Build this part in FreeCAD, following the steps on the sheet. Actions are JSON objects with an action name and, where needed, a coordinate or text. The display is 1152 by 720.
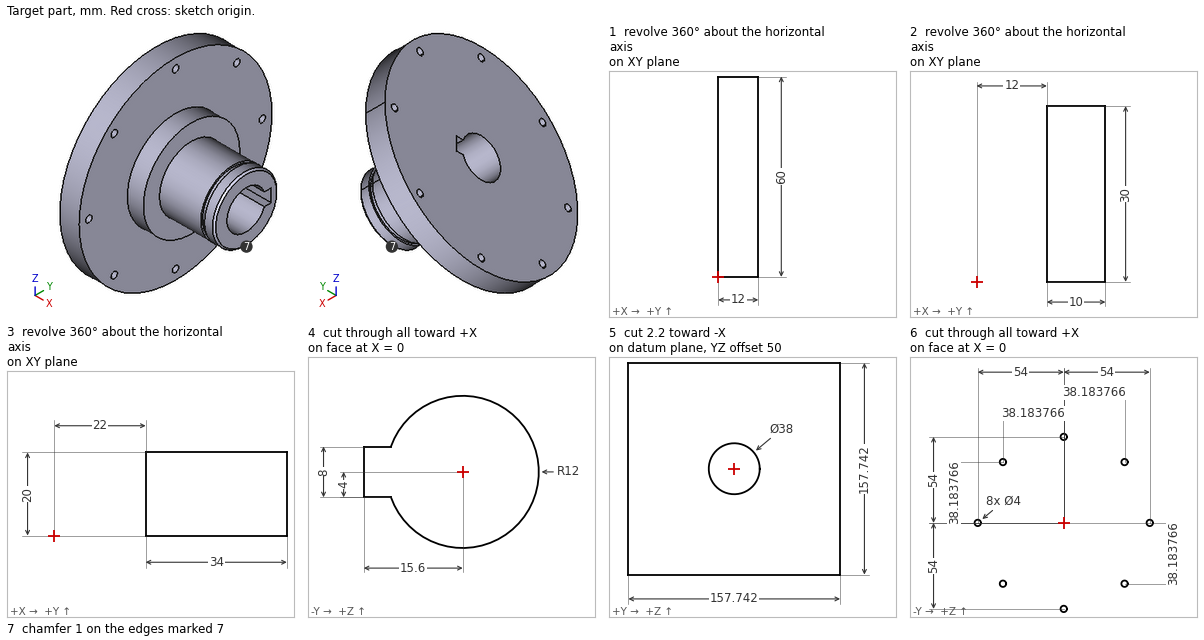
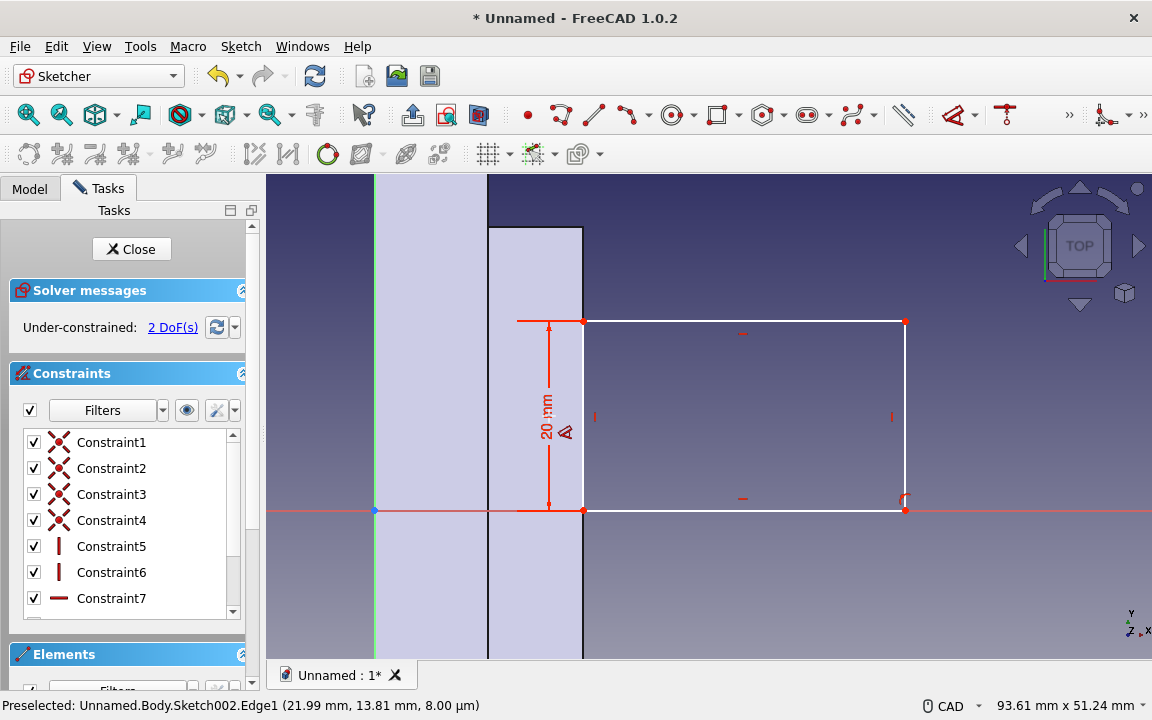
{"action": "left_click", "coordinate": [680, 511]}
{"action": "left_click", "coordinate": [744, 545]}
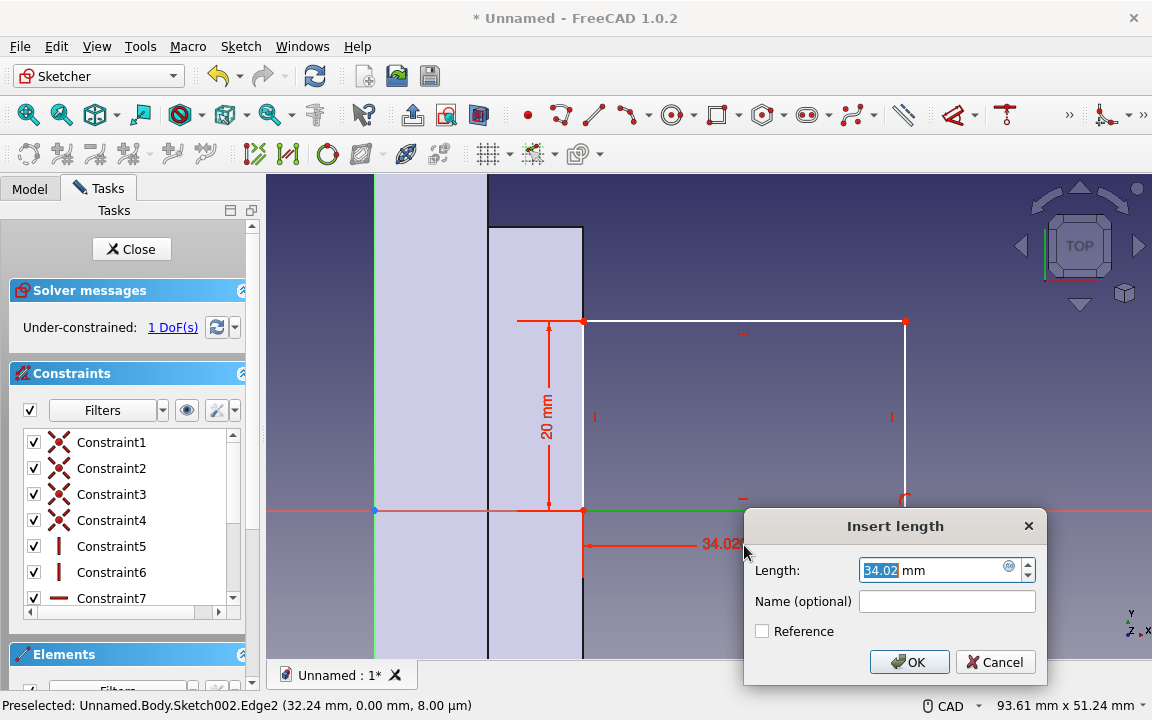
{"action": "type", "text": "34"}
{"action": "key", "text": "Return"}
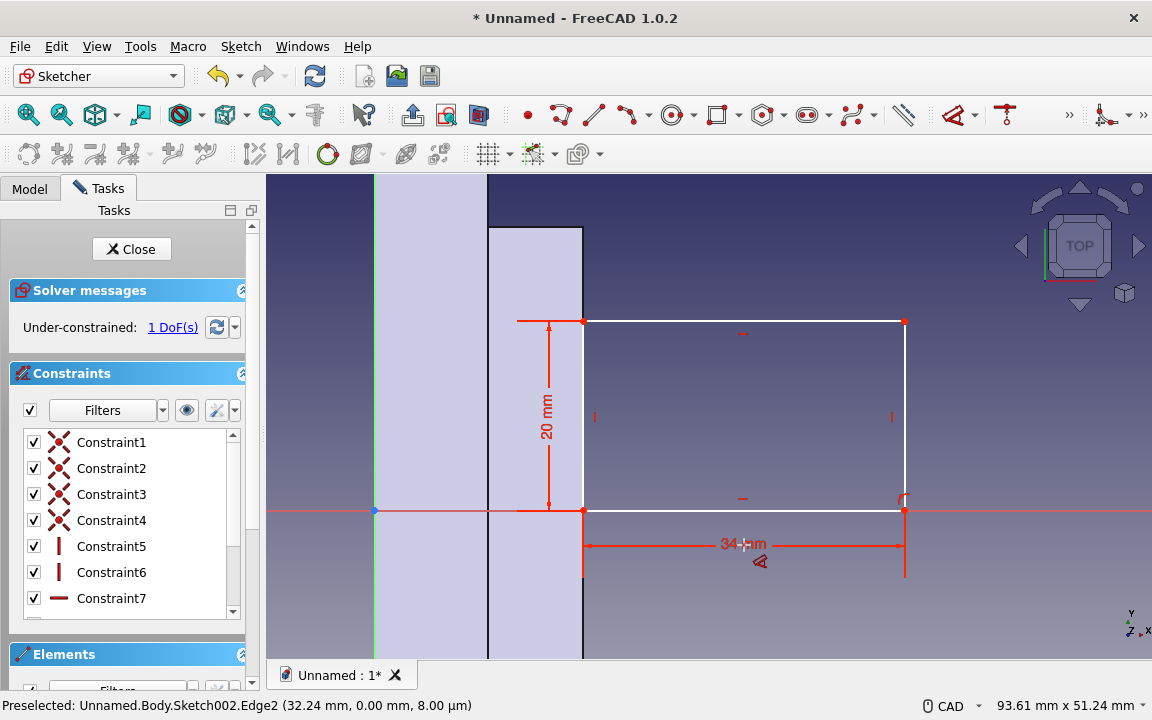
{"action": "left_click", "coordinate": [583, 321]}
{"action": "left_click", "coordinate": [479, 545]}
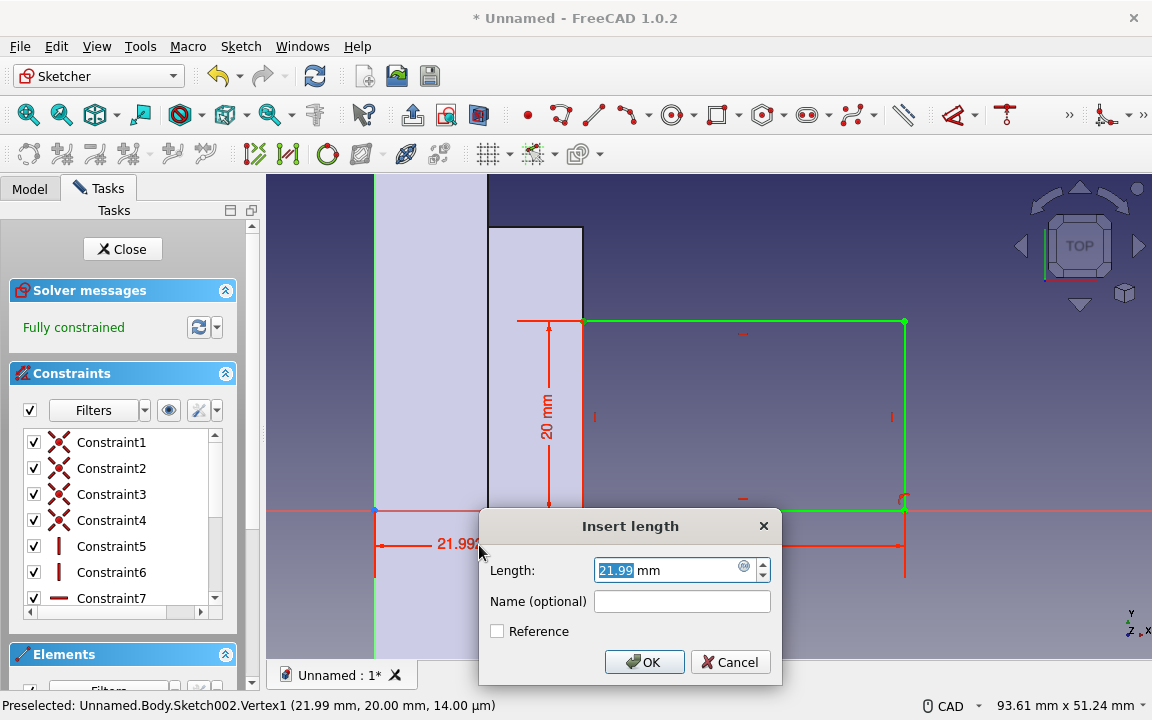
{"action": "type", "text": "22"}
{"action": "key", "text": "Return"}
{"action": "key", "text": "Escape"}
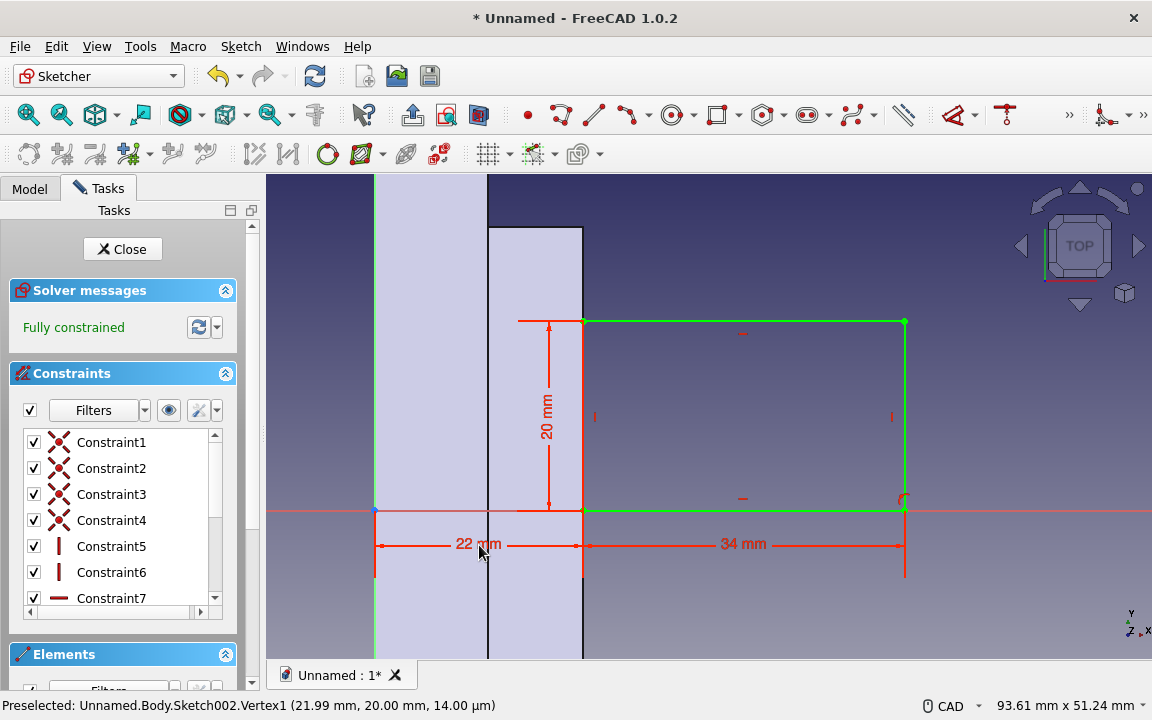
{"action": "left_click", "coordinate": [123, 249]}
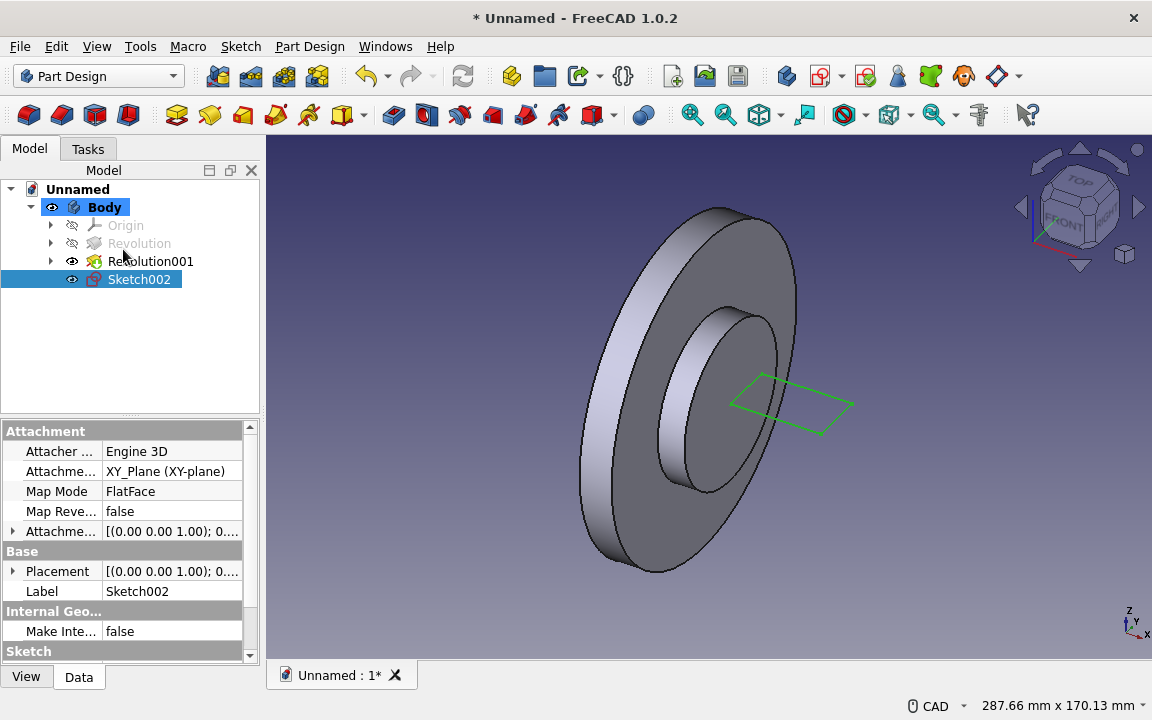
{"action": "left_click", "coordinate": [210, 116]}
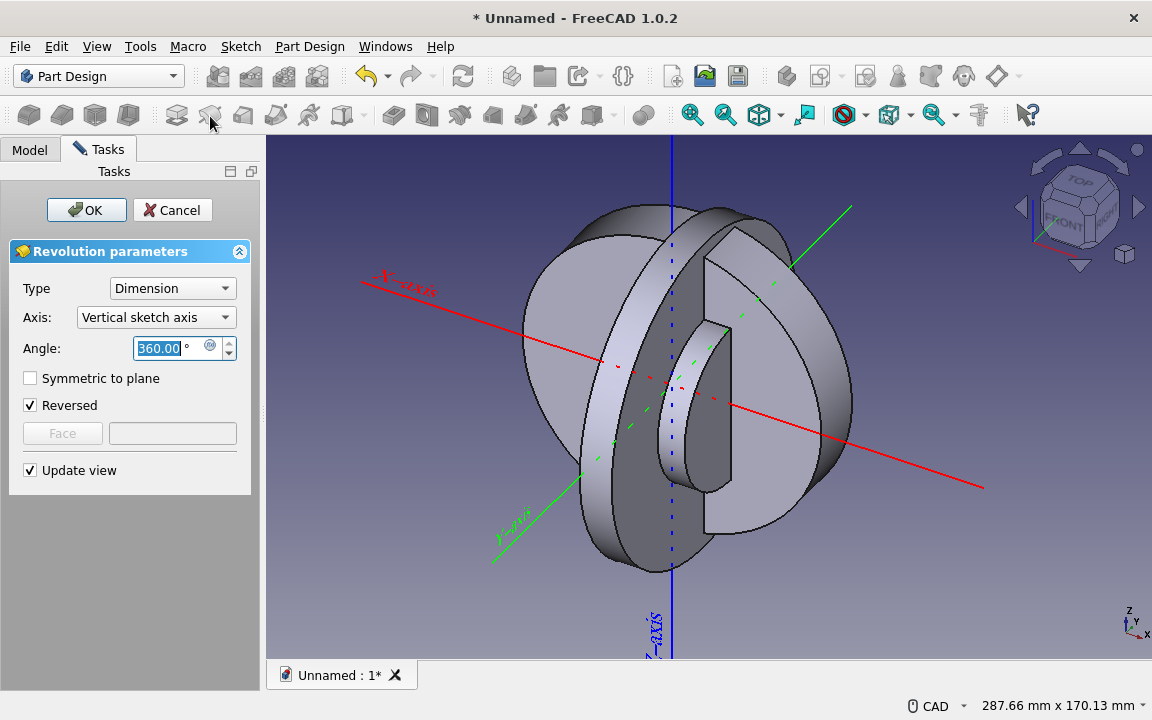
{"action": "left_click", "coordinate": [157, 318]}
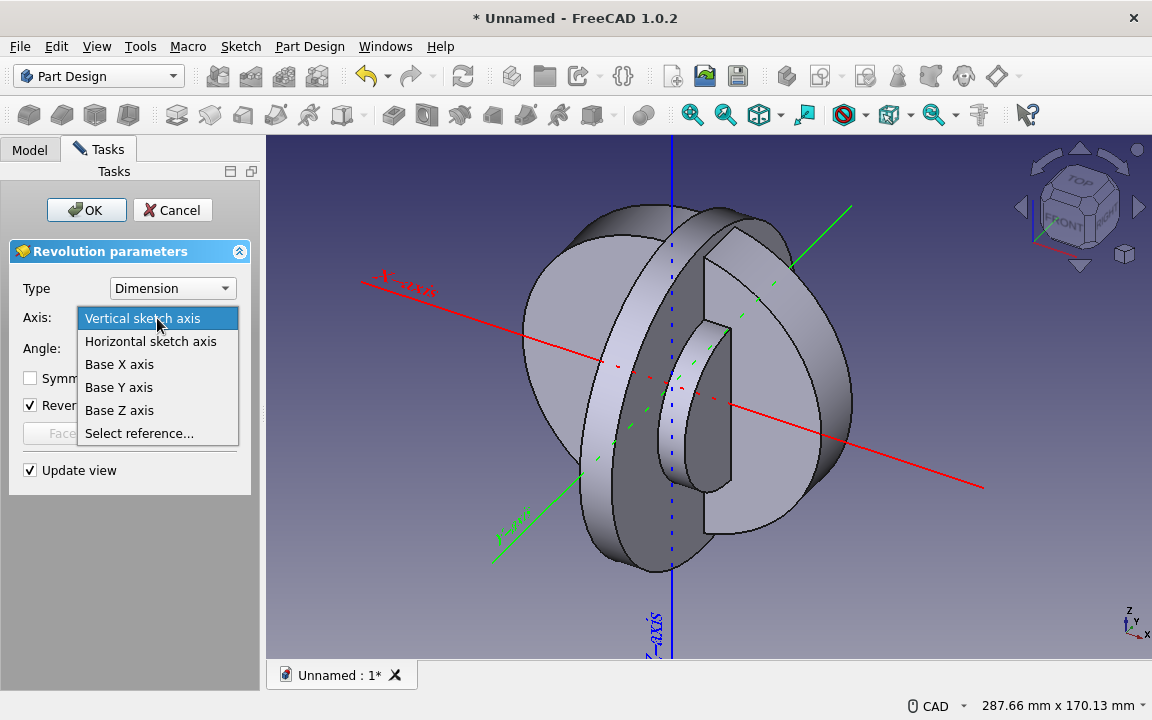
{"action": "left_click", "coordinate": [156, 342]}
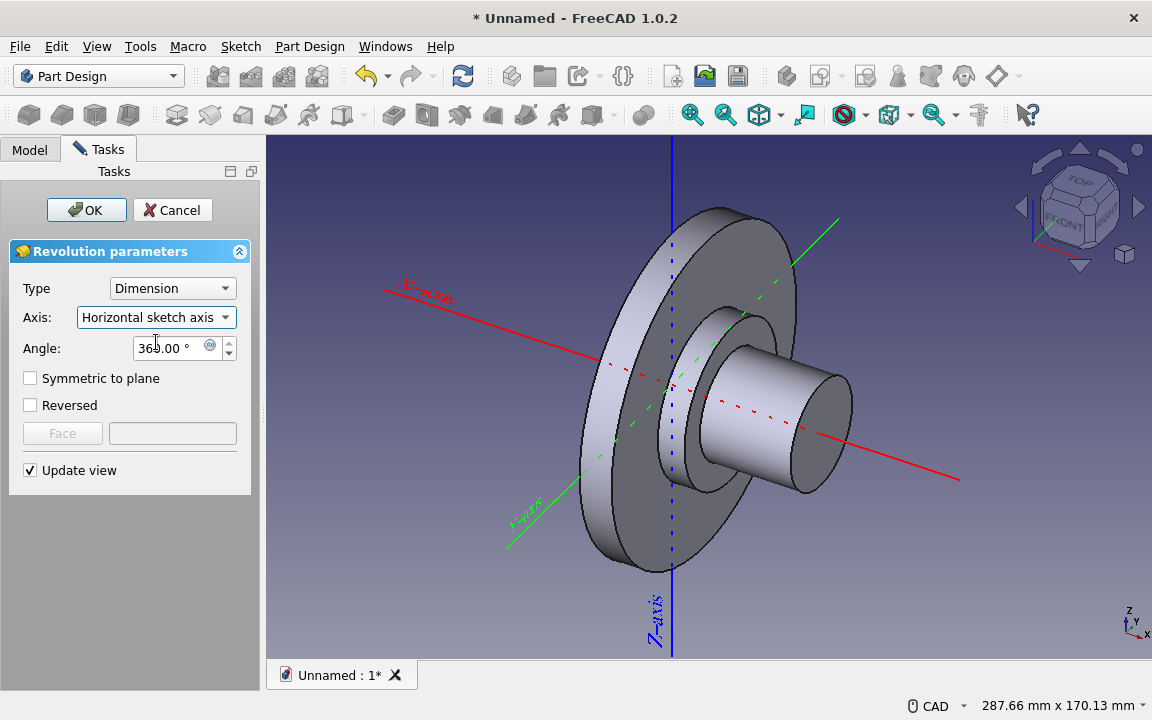
{"action": "left_click", "coordinate": [87, 210]}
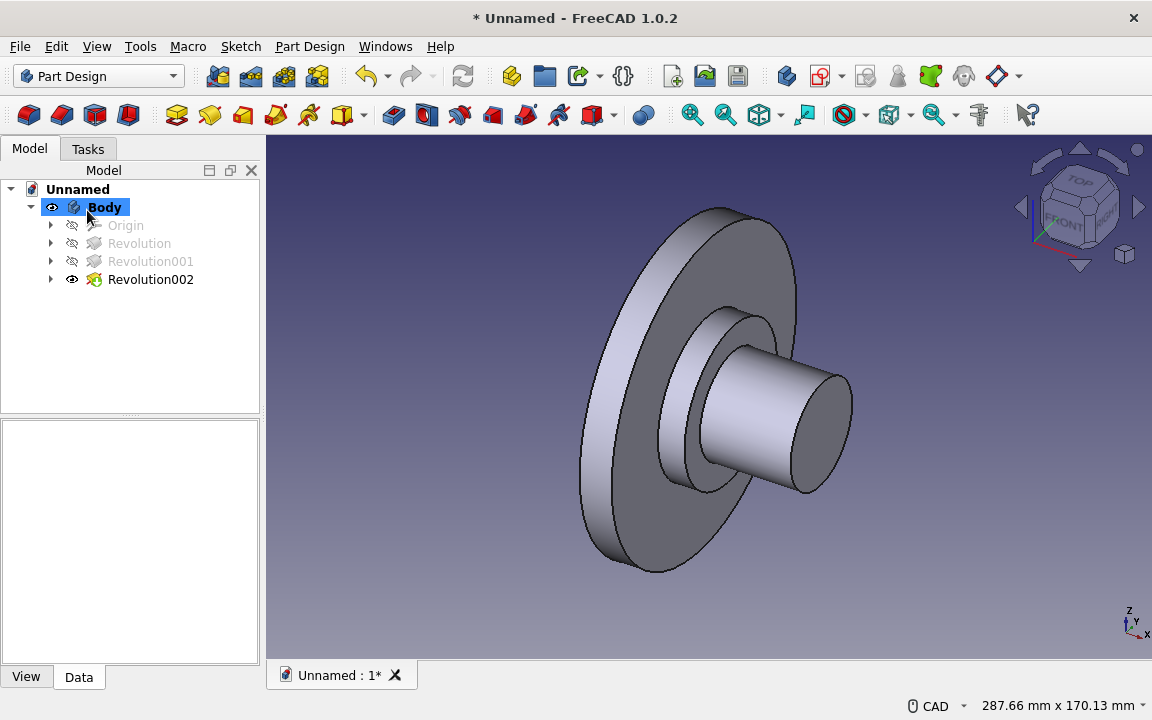
{"action": "left_click", "coordinate": [693, 116]}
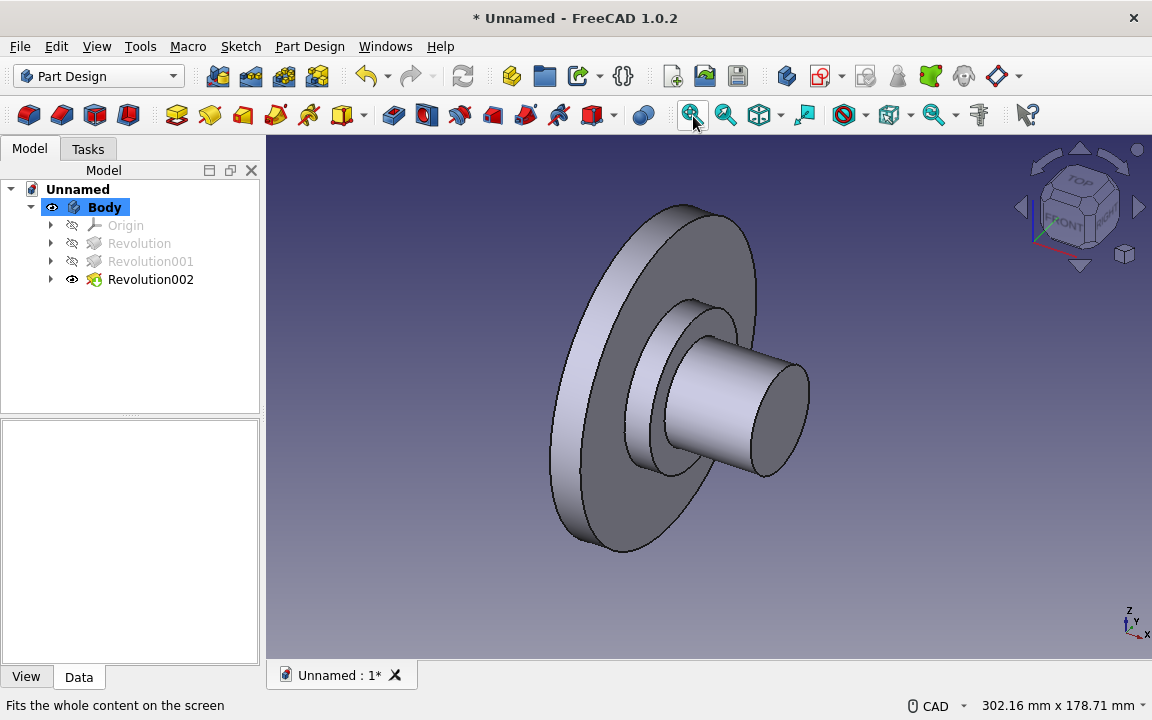
{"action": "key", "text": "6"}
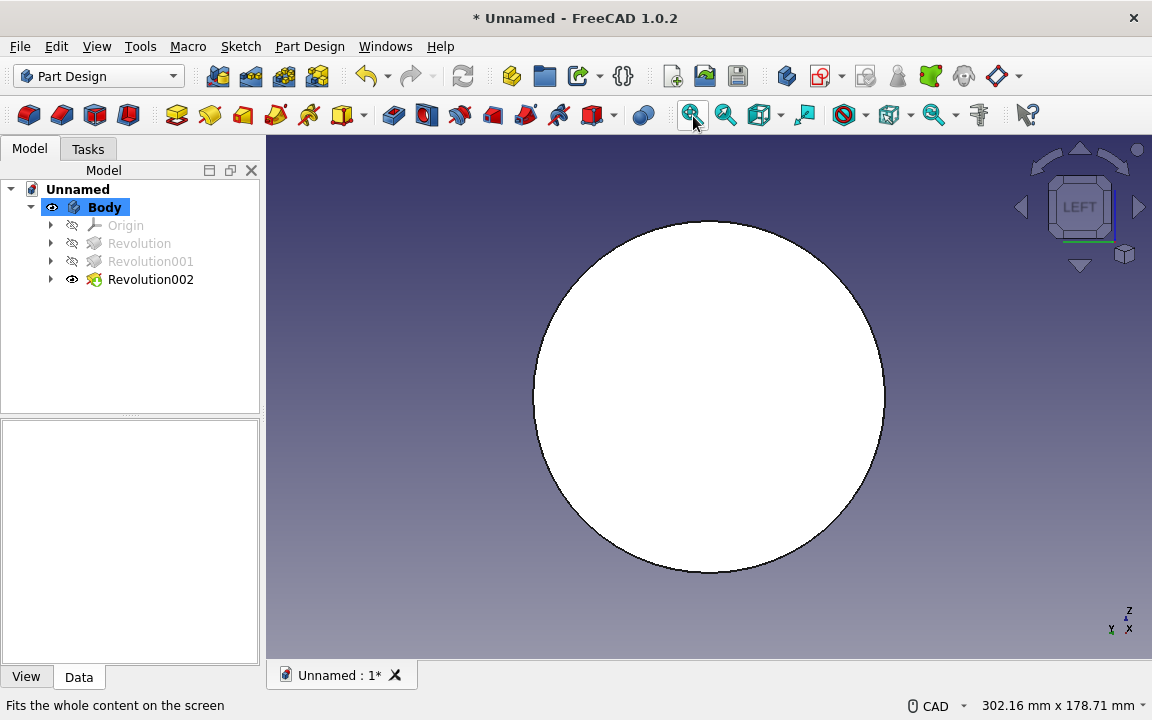
{"action": "left_click", "coordinate": [709, 396]}